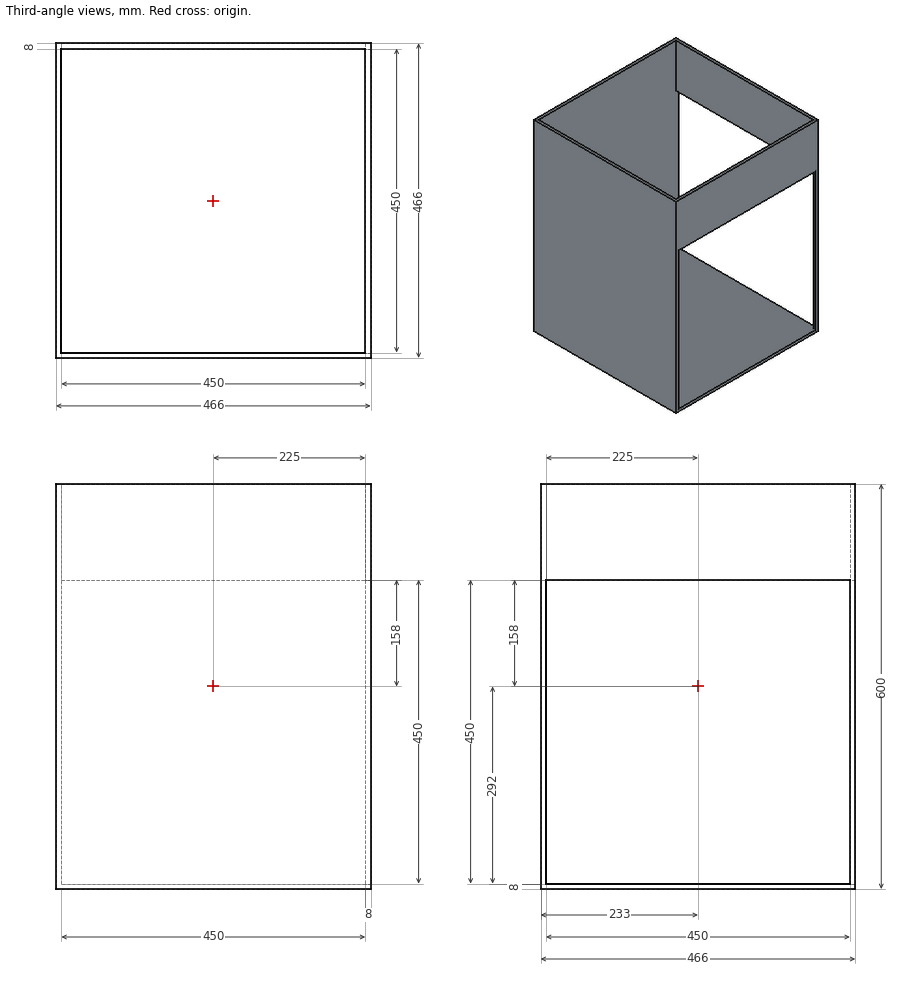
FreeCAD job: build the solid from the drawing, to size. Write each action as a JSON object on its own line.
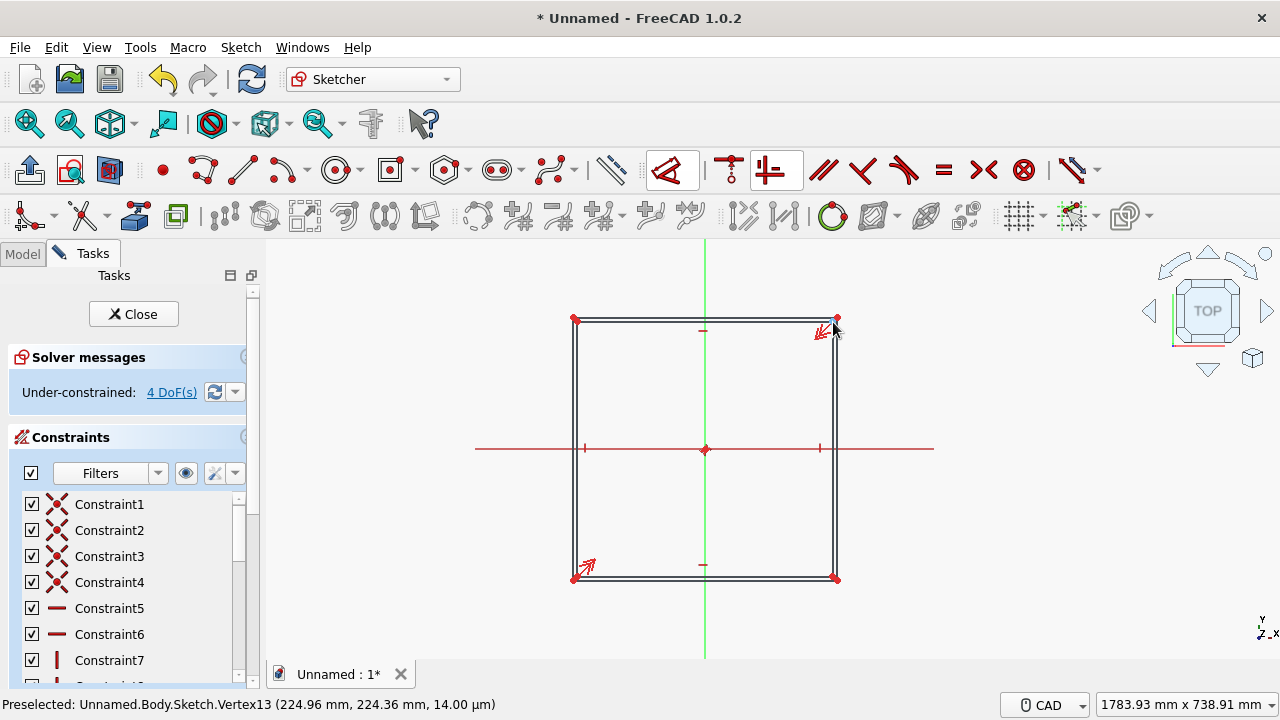
{"action": "scroll", "coordinate": [652, 581], "scroll_direction": "up", "scroll_amount": 7}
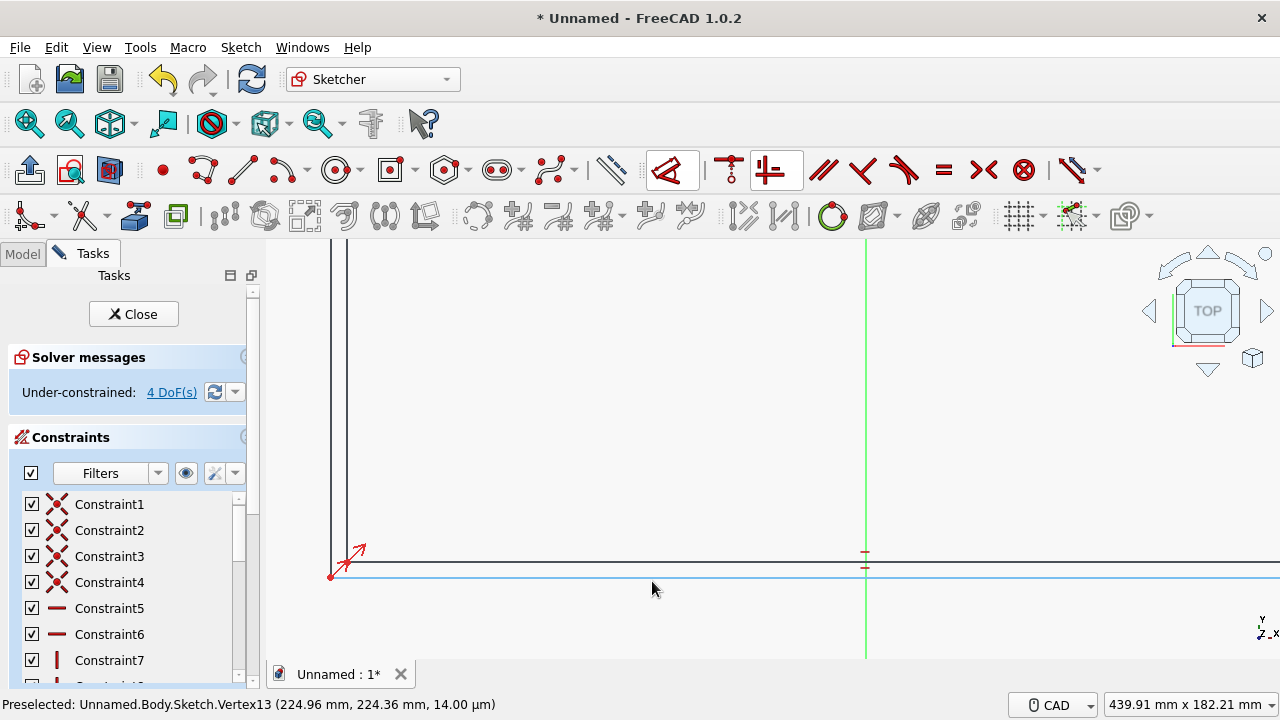
{"action": "left_click", "coordinate": [652, 578]}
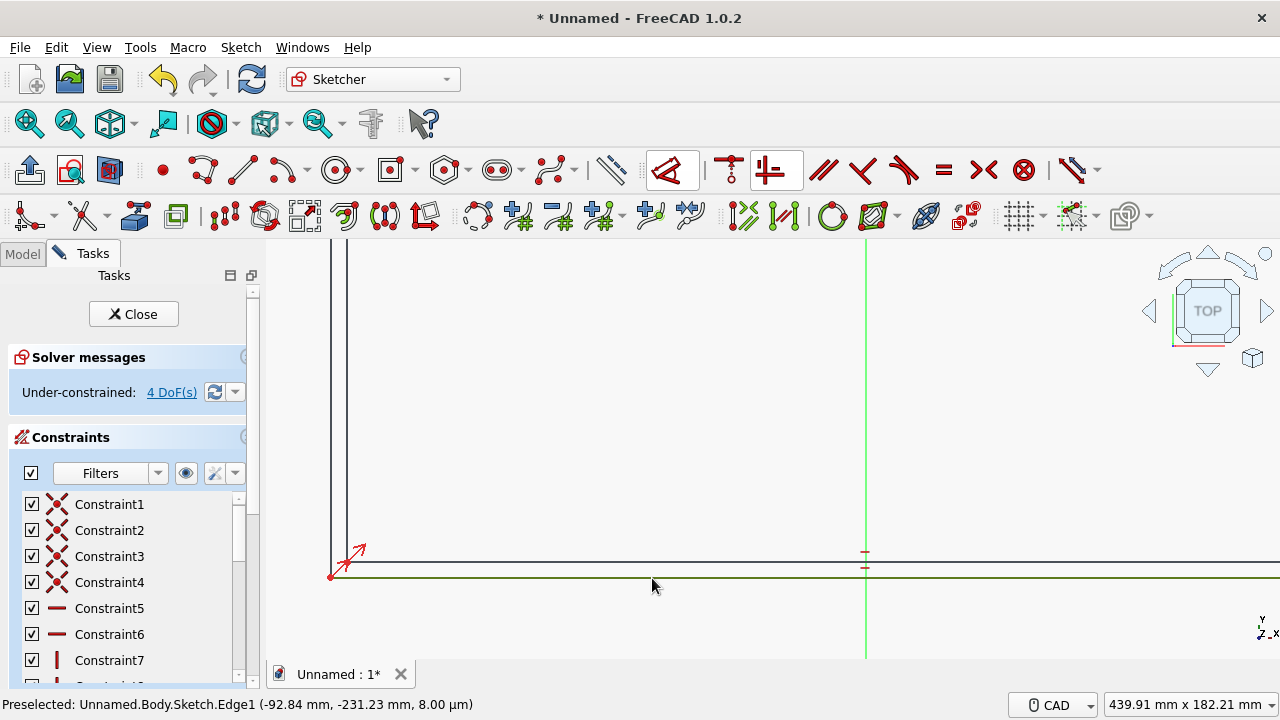
{"action": "left_click", "coordinate": [694, 170]}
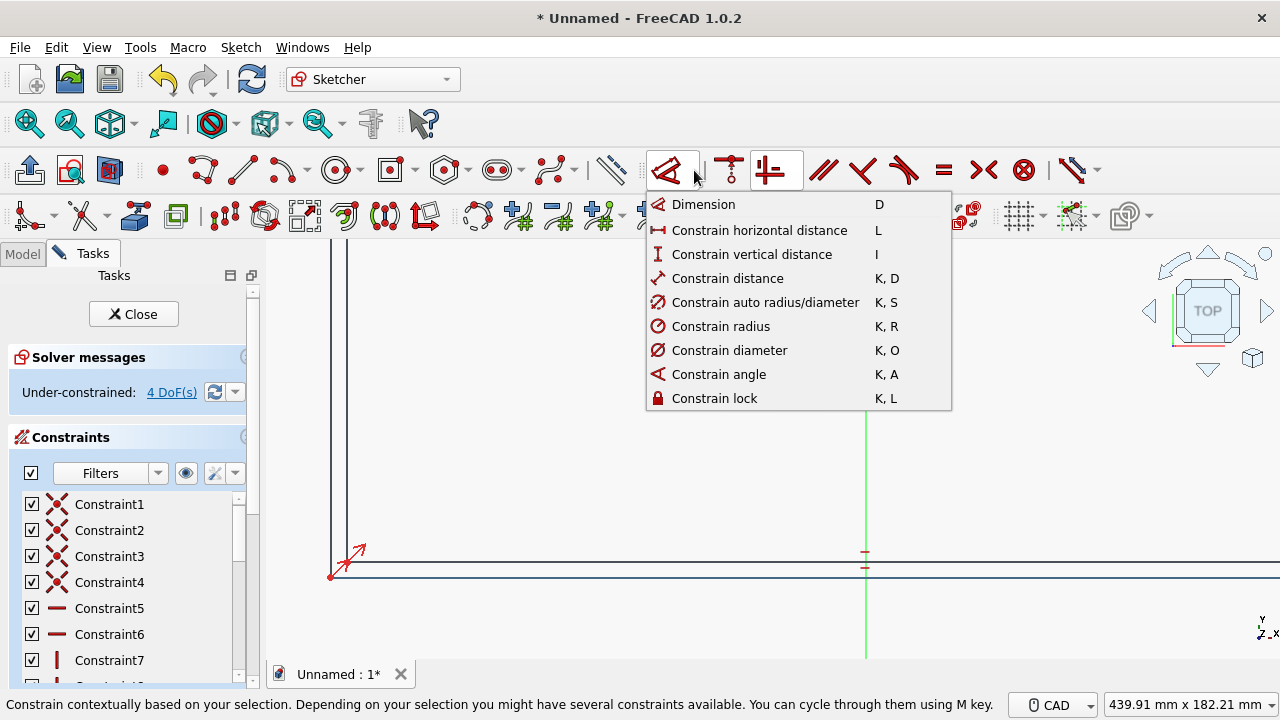
{"action": "left_click", "coordinate": [799, 230]}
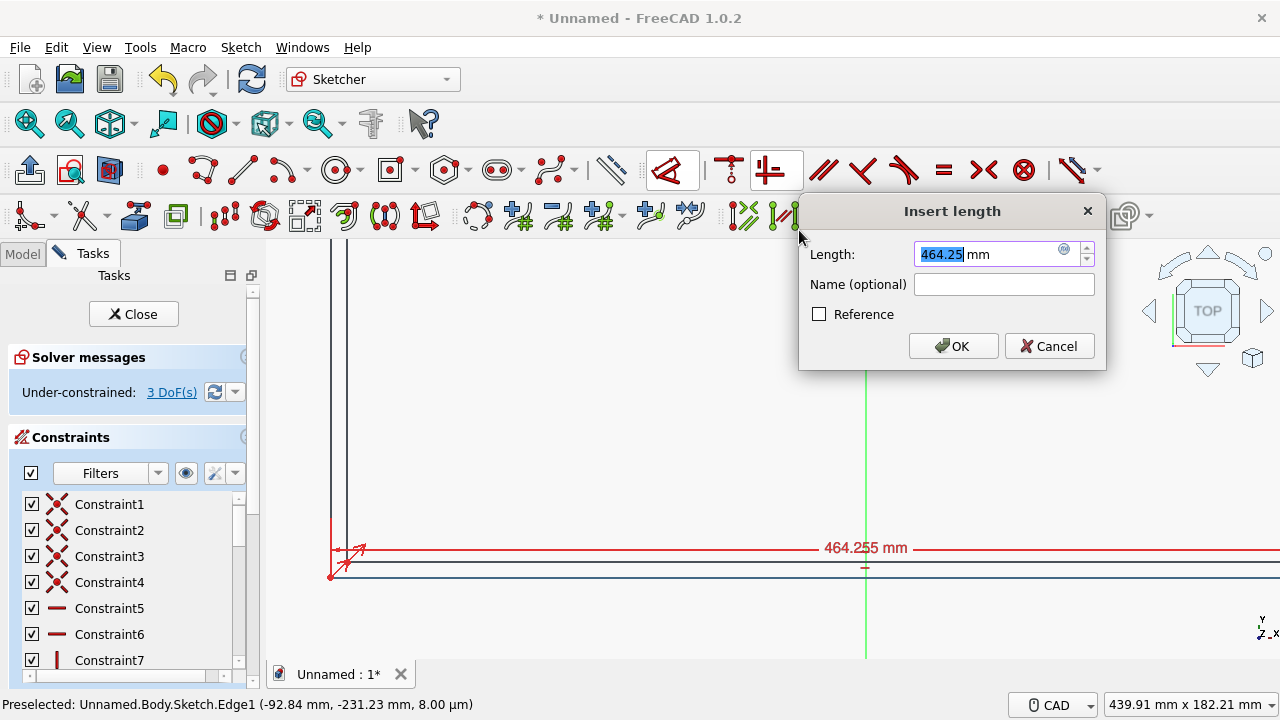
{"action": "type", "text": "466"}
{"action": "key", "text": "Return"}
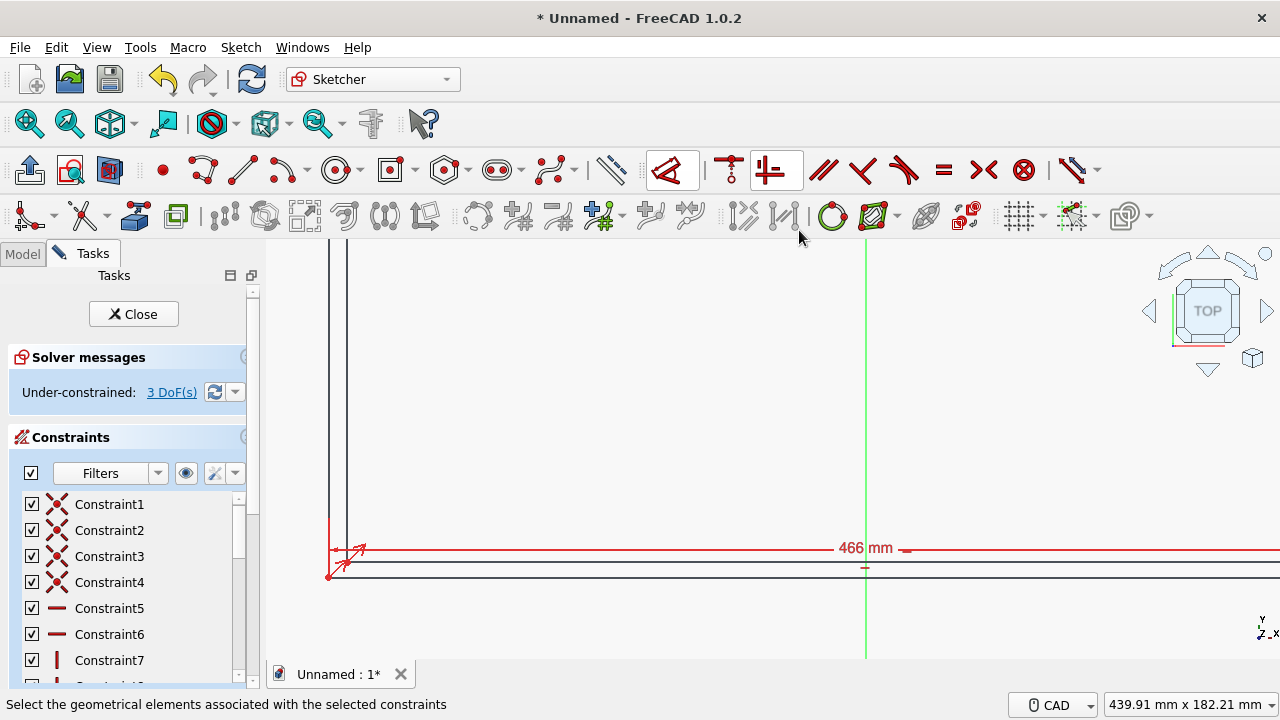
{"action": "scroll", "coordinate": [652, 581], "scroll_direction": "down", "scroll_amount": 7}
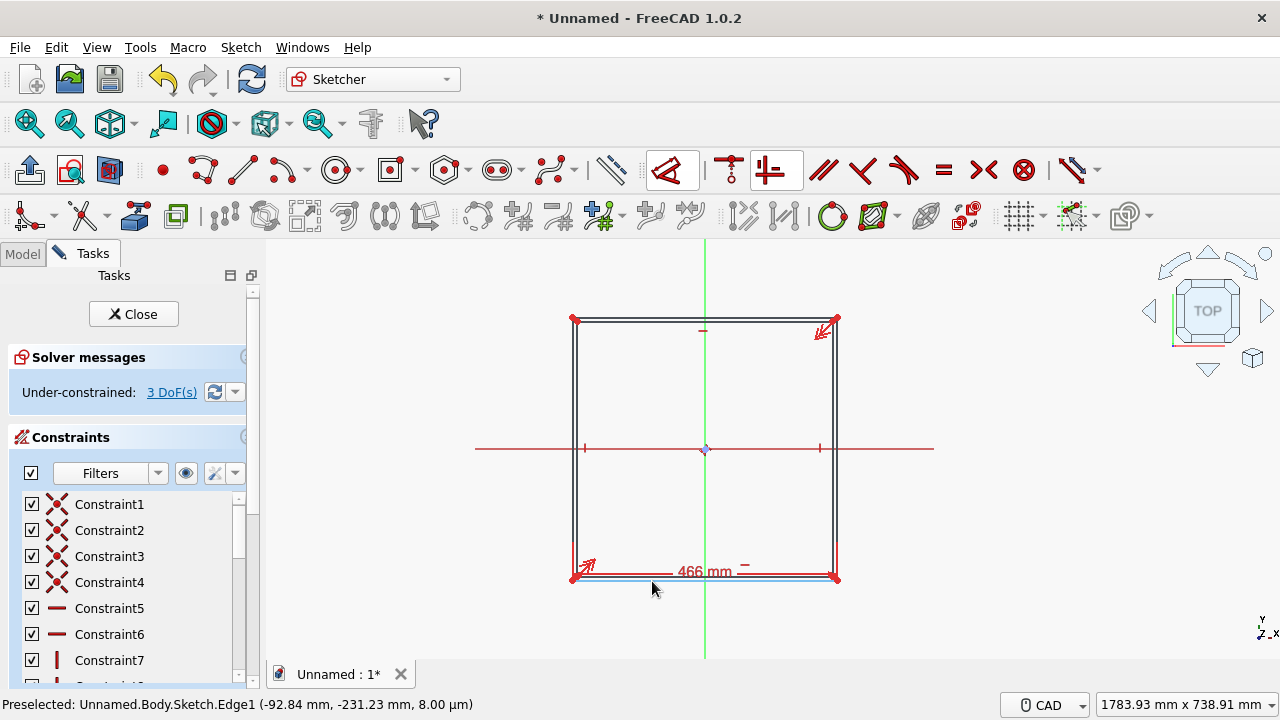
{"action": "scroll", "coordinate": [837, 502], "scroll_direction": "up", "scroll_amount": 6}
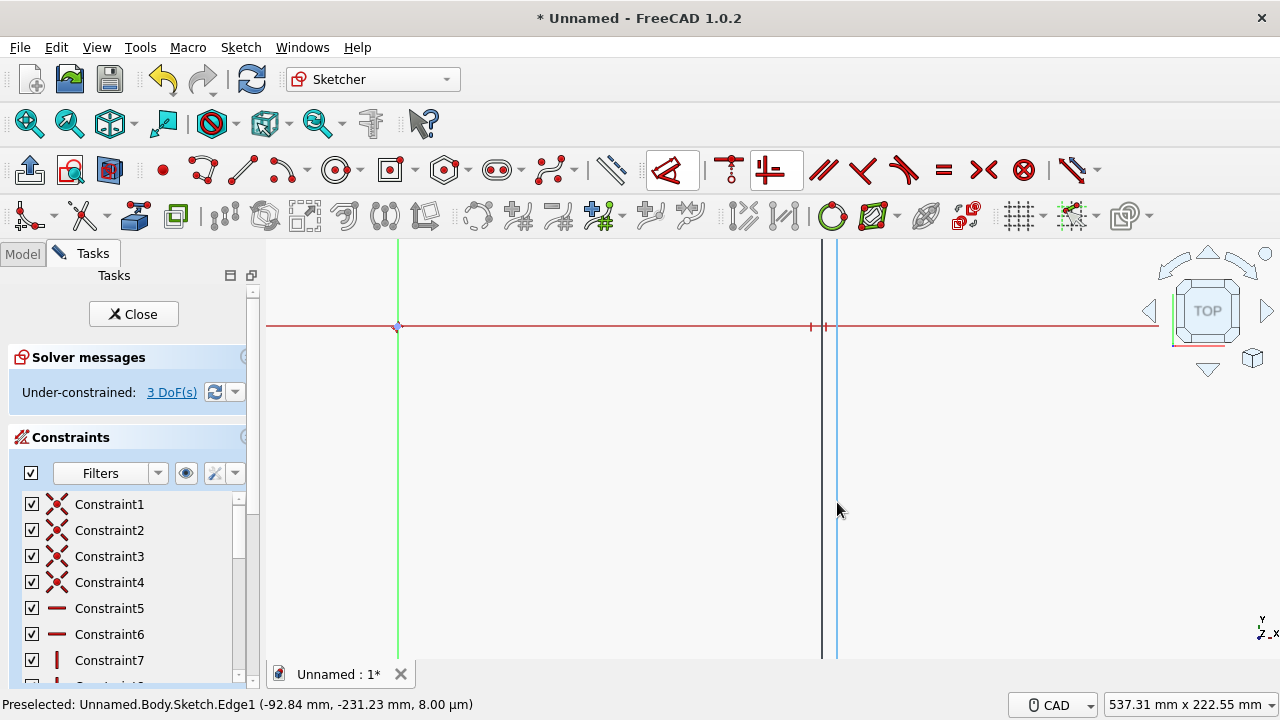
{"action": "left_click", "coordinate": [837, 501]}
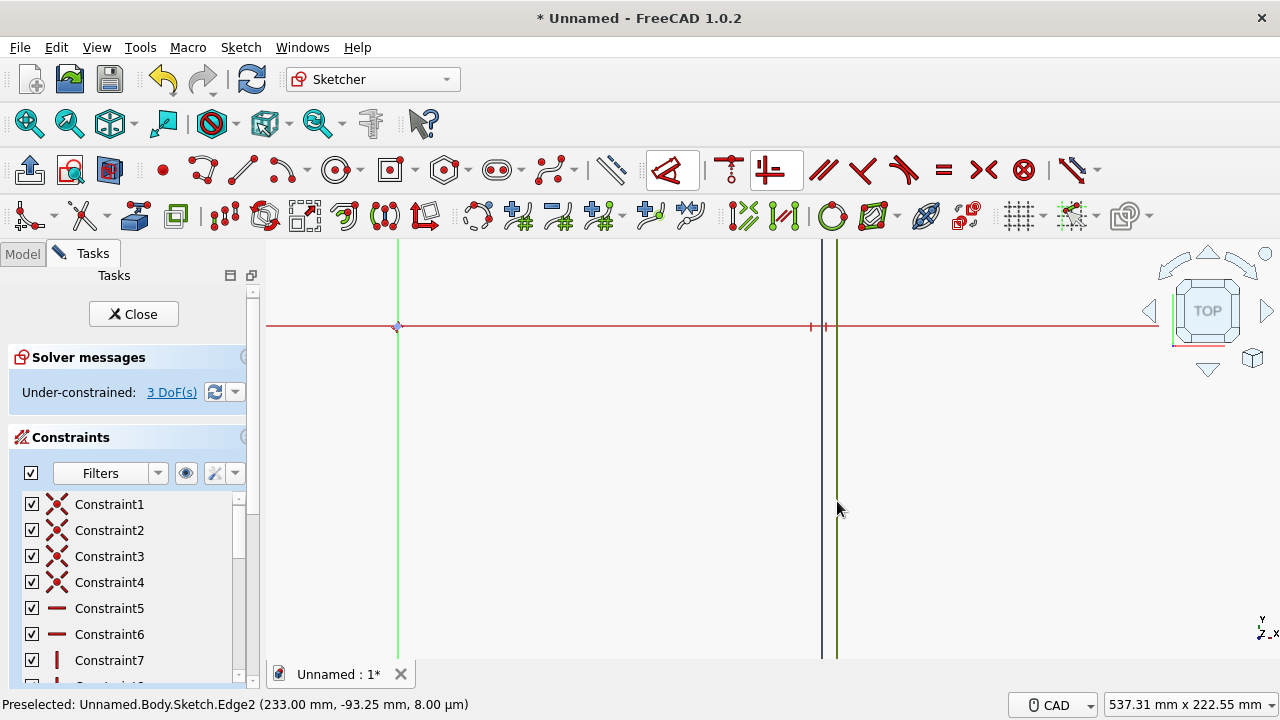
{"action": "left_click", "coordinate": [694, 170]}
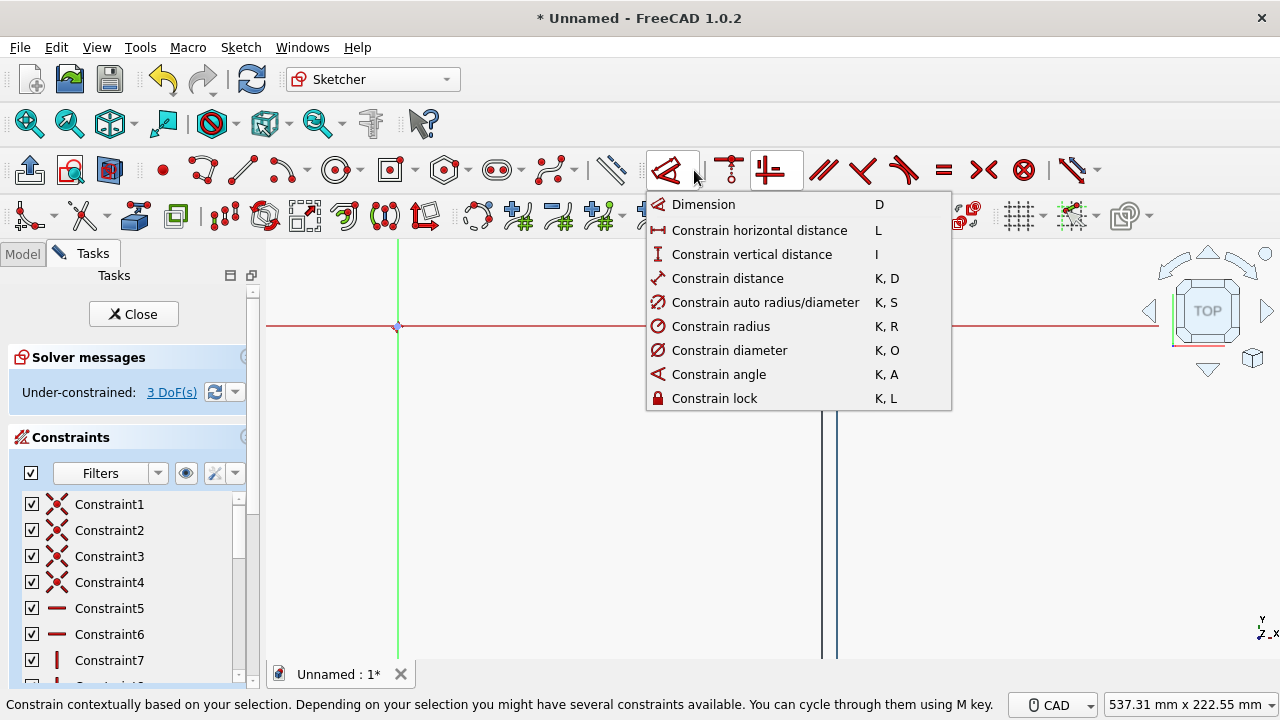
{"action": "left_click", "coordinate": [799, 254]}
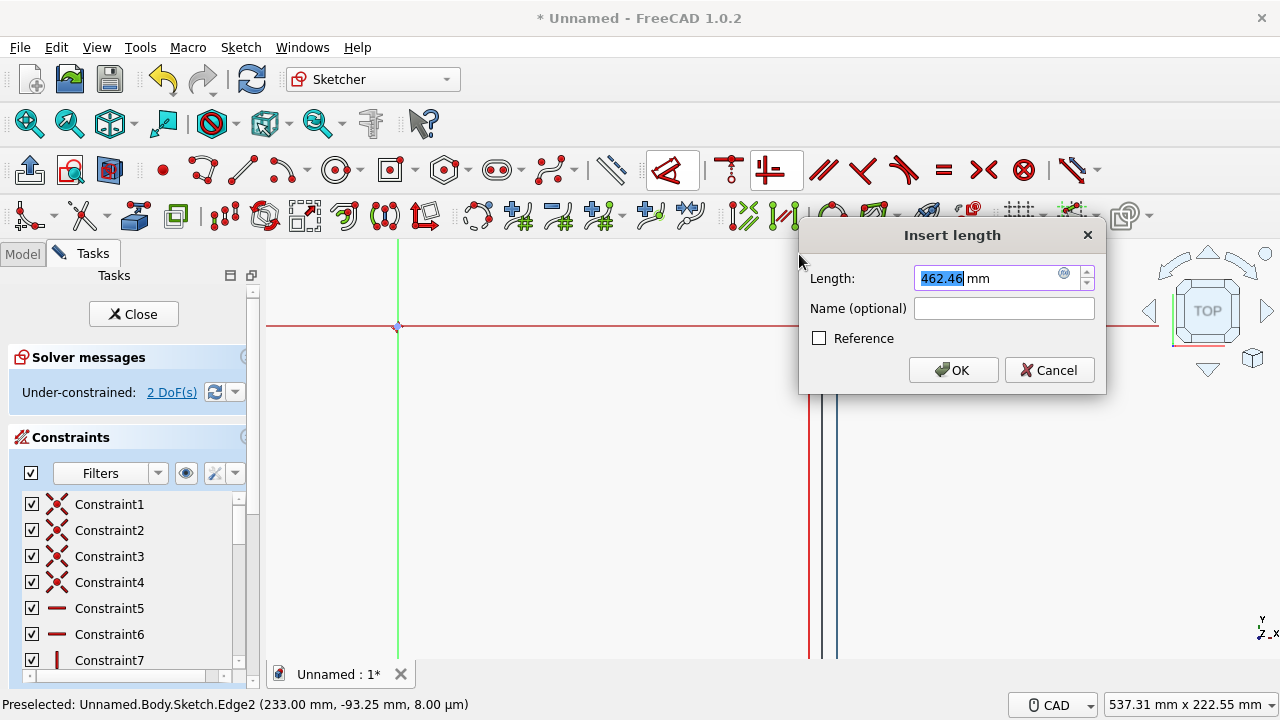
{"action": "type", "text": "466"}
{"action": "key", "text": "Return"}